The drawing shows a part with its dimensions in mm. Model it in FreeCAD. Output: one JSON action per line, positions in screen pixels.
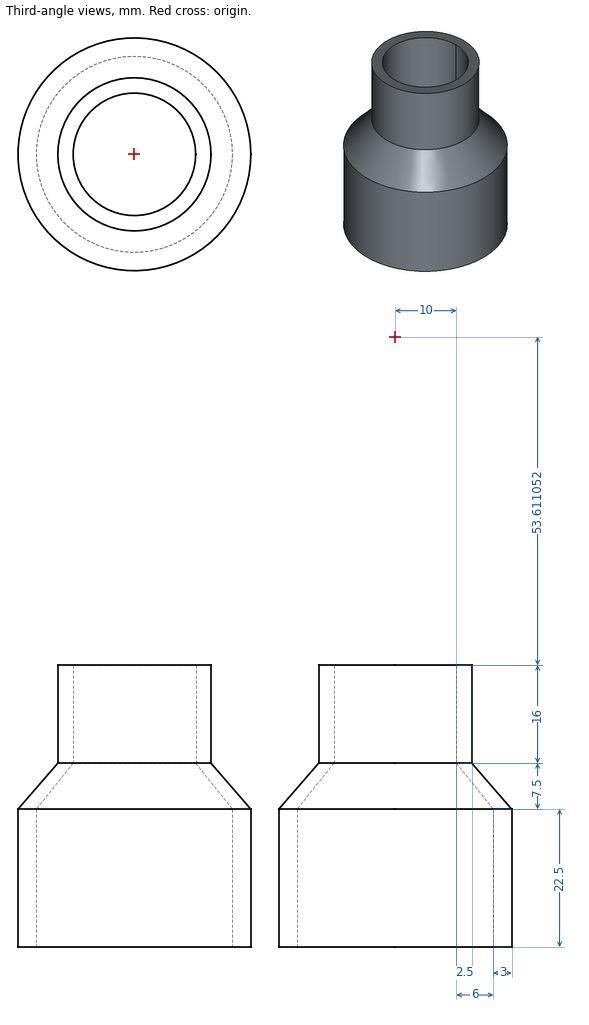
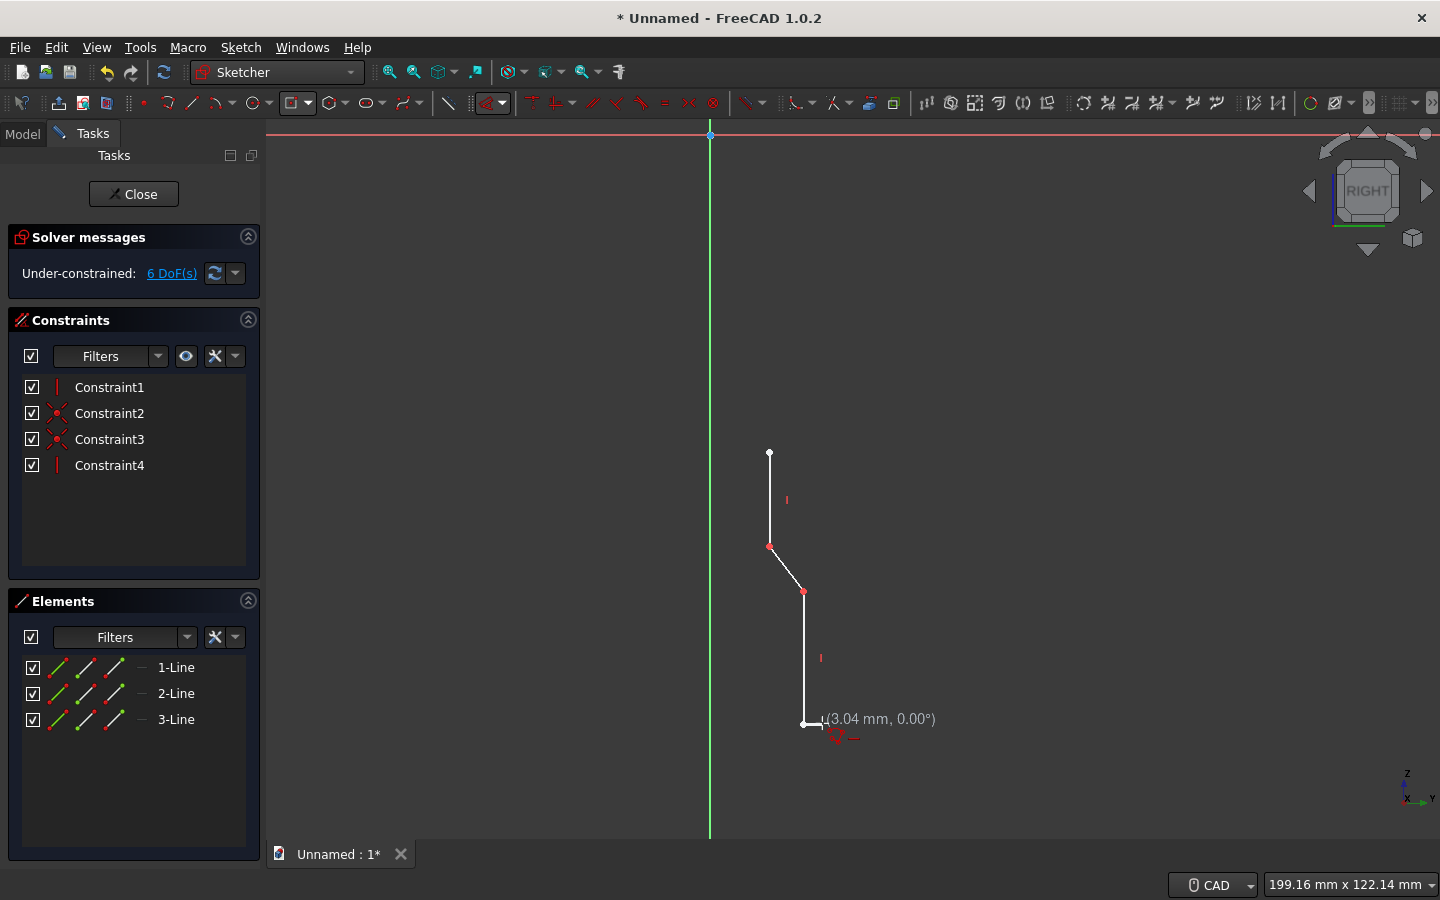
{"action": "left_click", "coordinate": [822, 723]}
{"action": "left_click", "coordinate": [822, 590]}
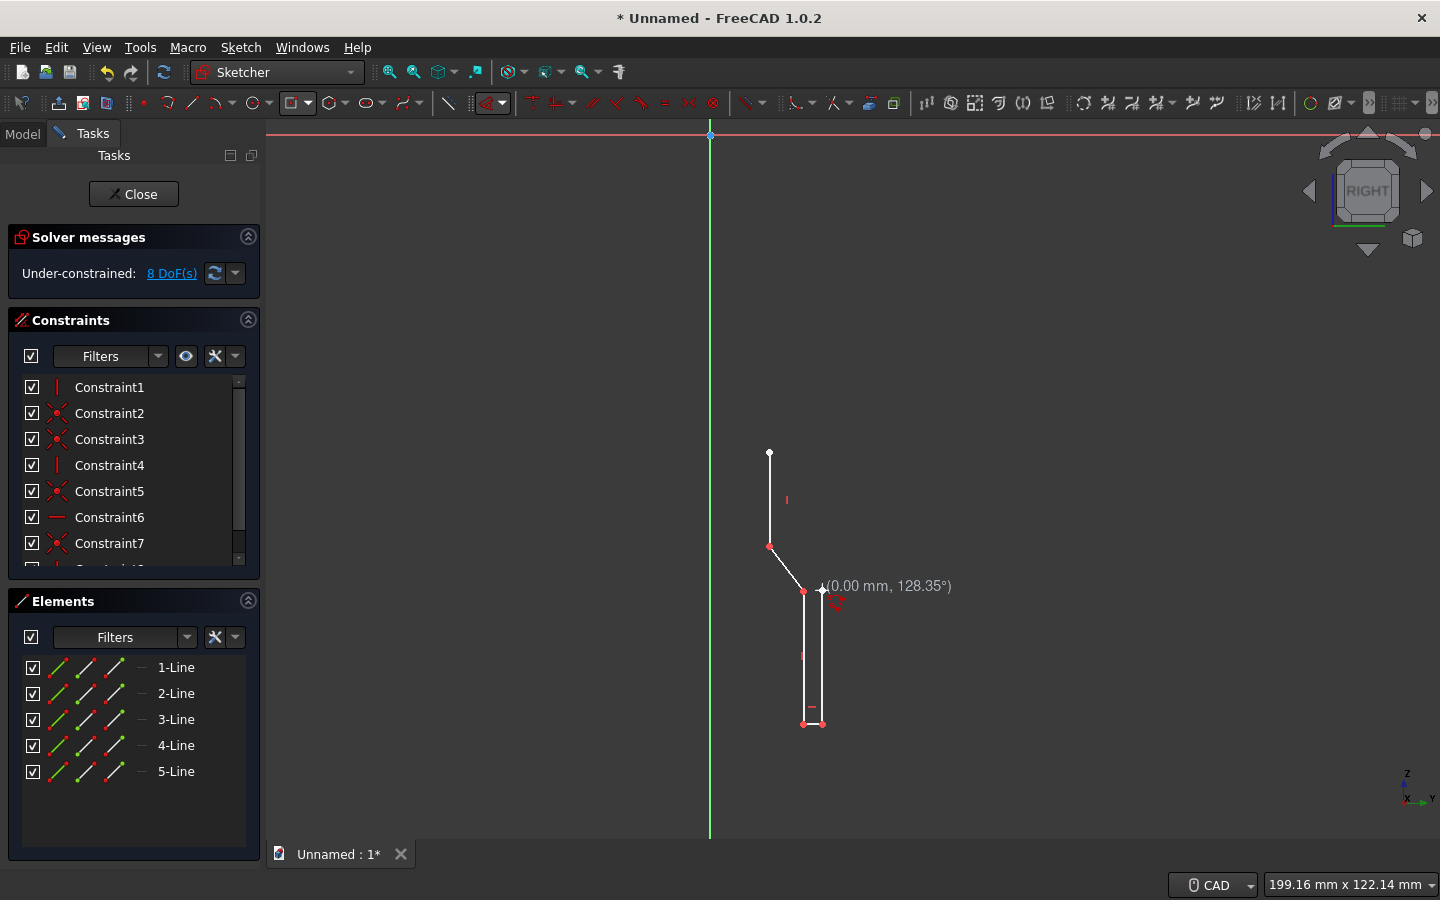
{"action": "scroll", "coordinate": [784, 545], "scroll_direction": "up", "scroll_amount": 2}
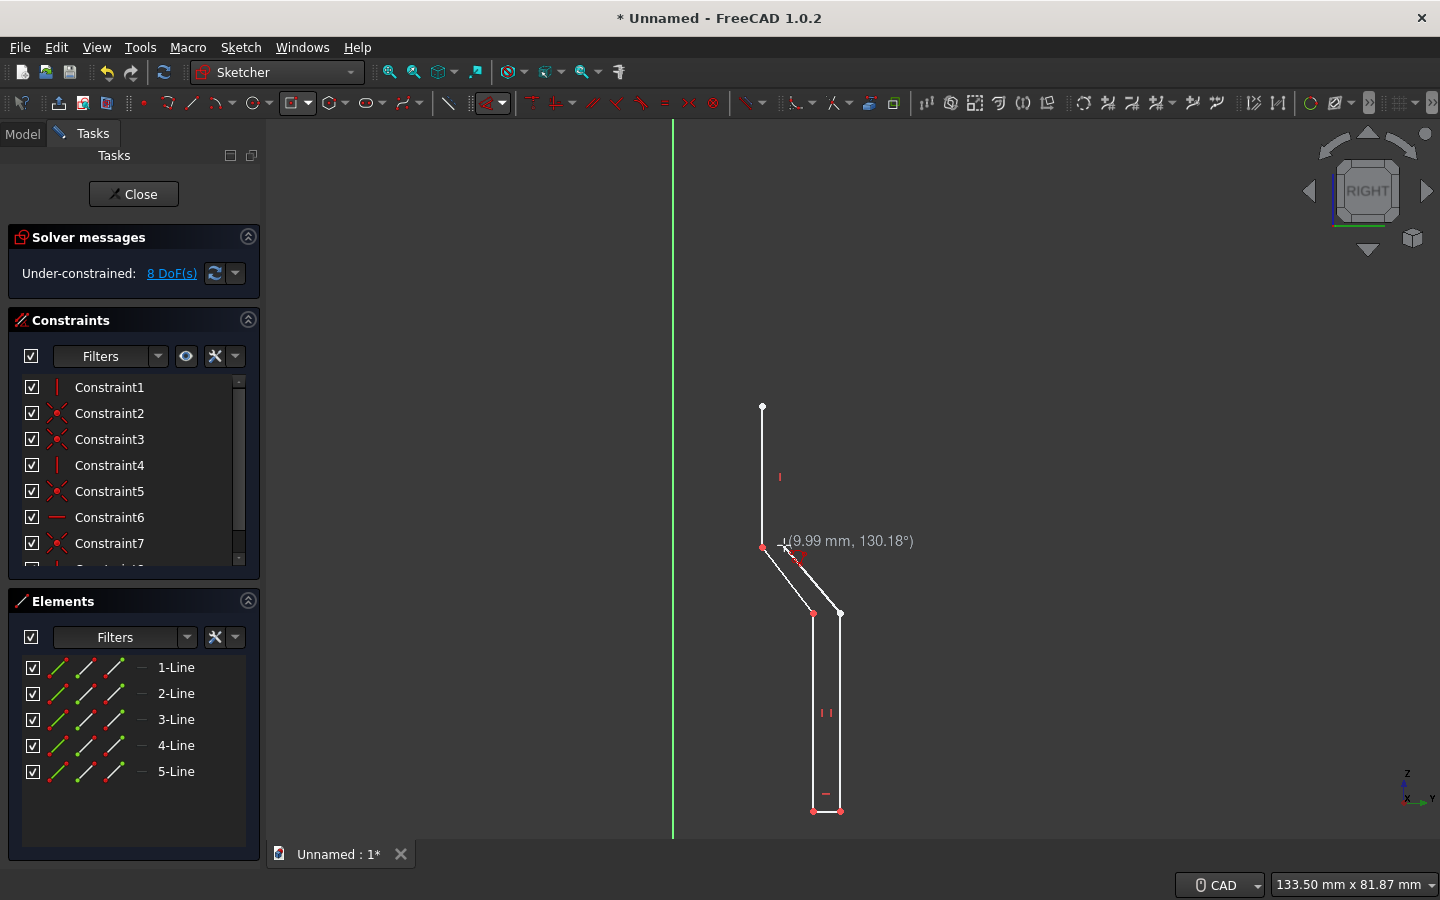
{"action": "left_click", "coordinate": [783, 545]}
{"action": "left_click", "coordinate": [783, 405]}
{"action": "left_click", "coordinate": [762, 407]}
{"action": "key", "text": "Escape"}
{"action": "key", "text": "Escape"}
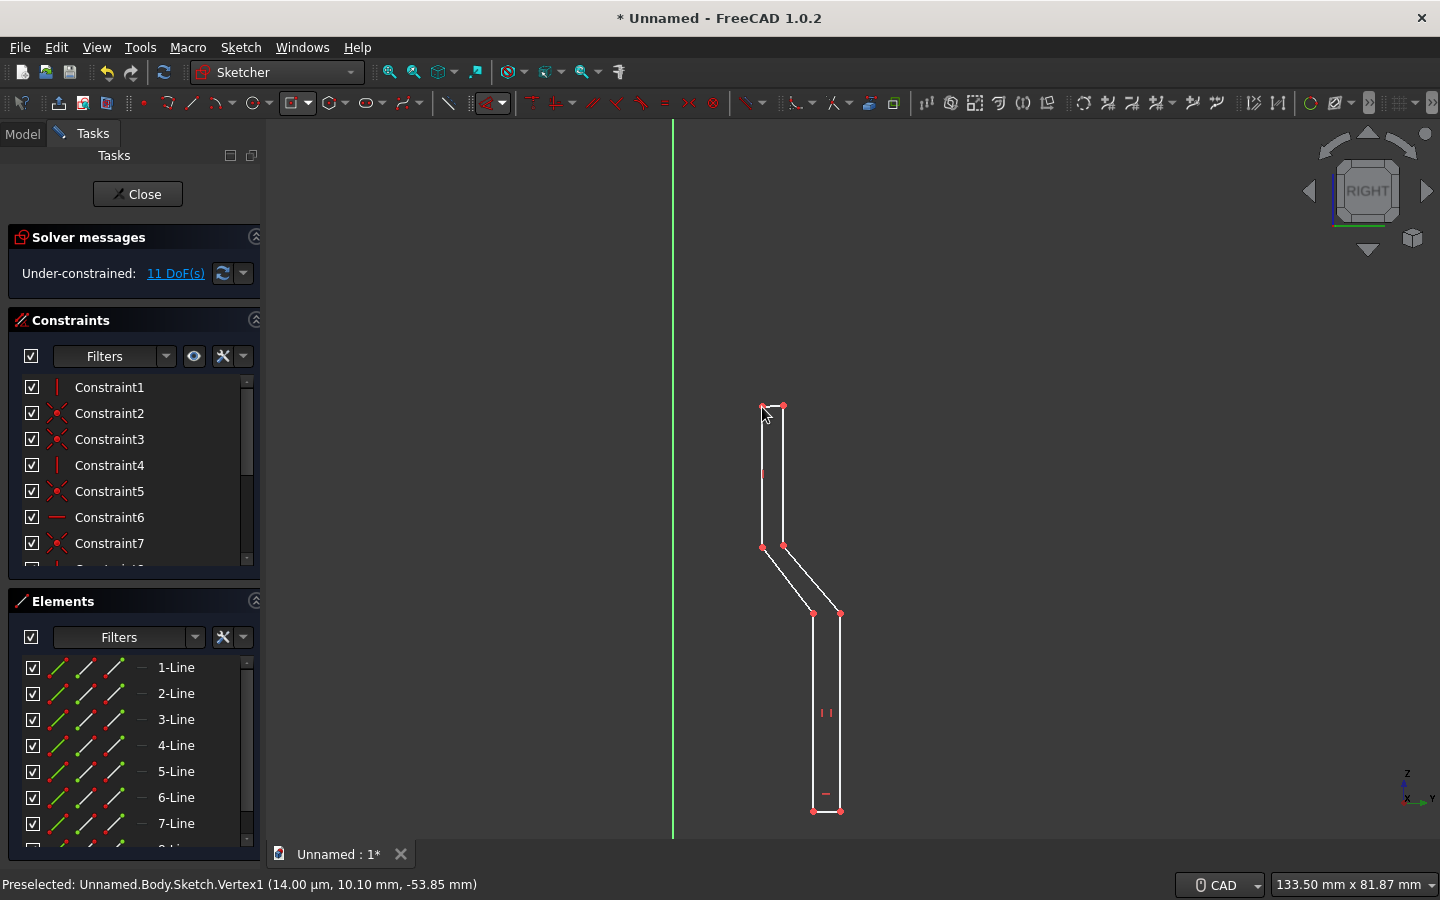
{"action": "scroll", "coordinate": [773, 406], "scroll_direction": "up", "scroll_amount": 2}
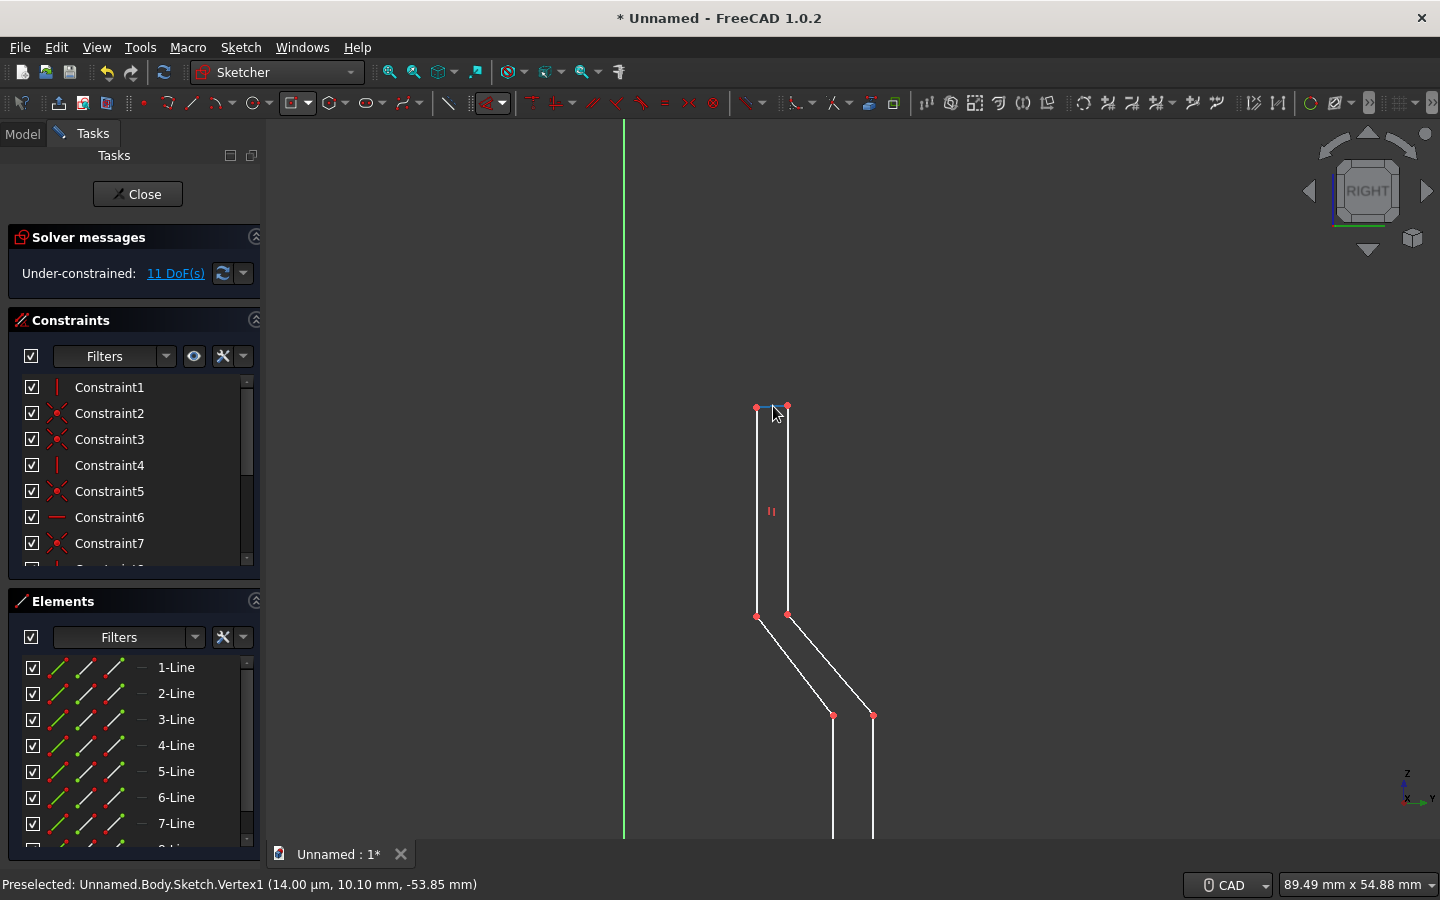
{"action": "left_click", "coordinate": [772, 406]}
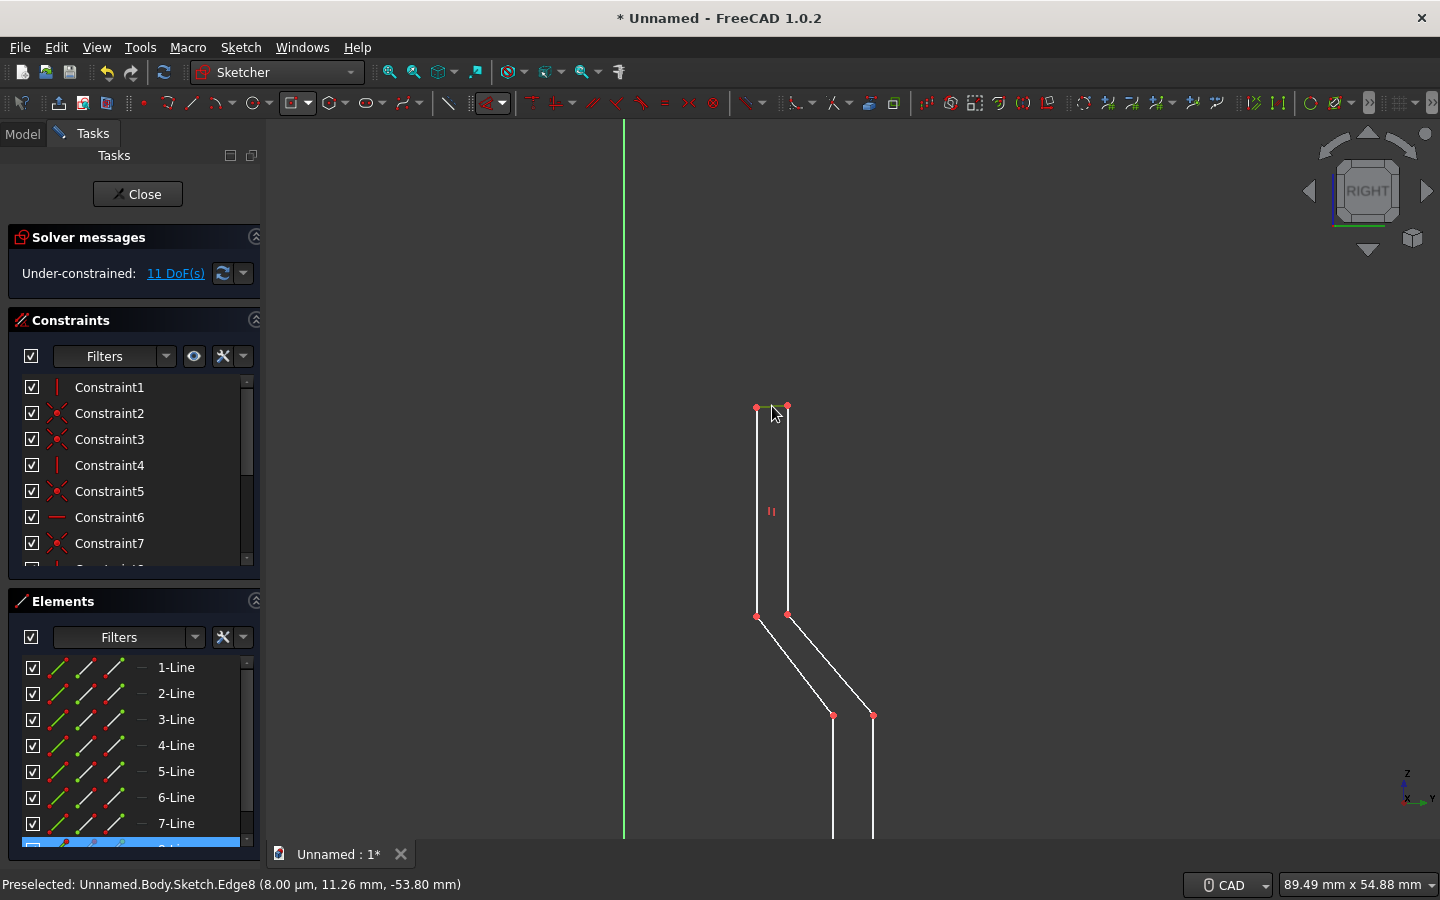
{"action": "left_click", "coordinate": [574, 104]}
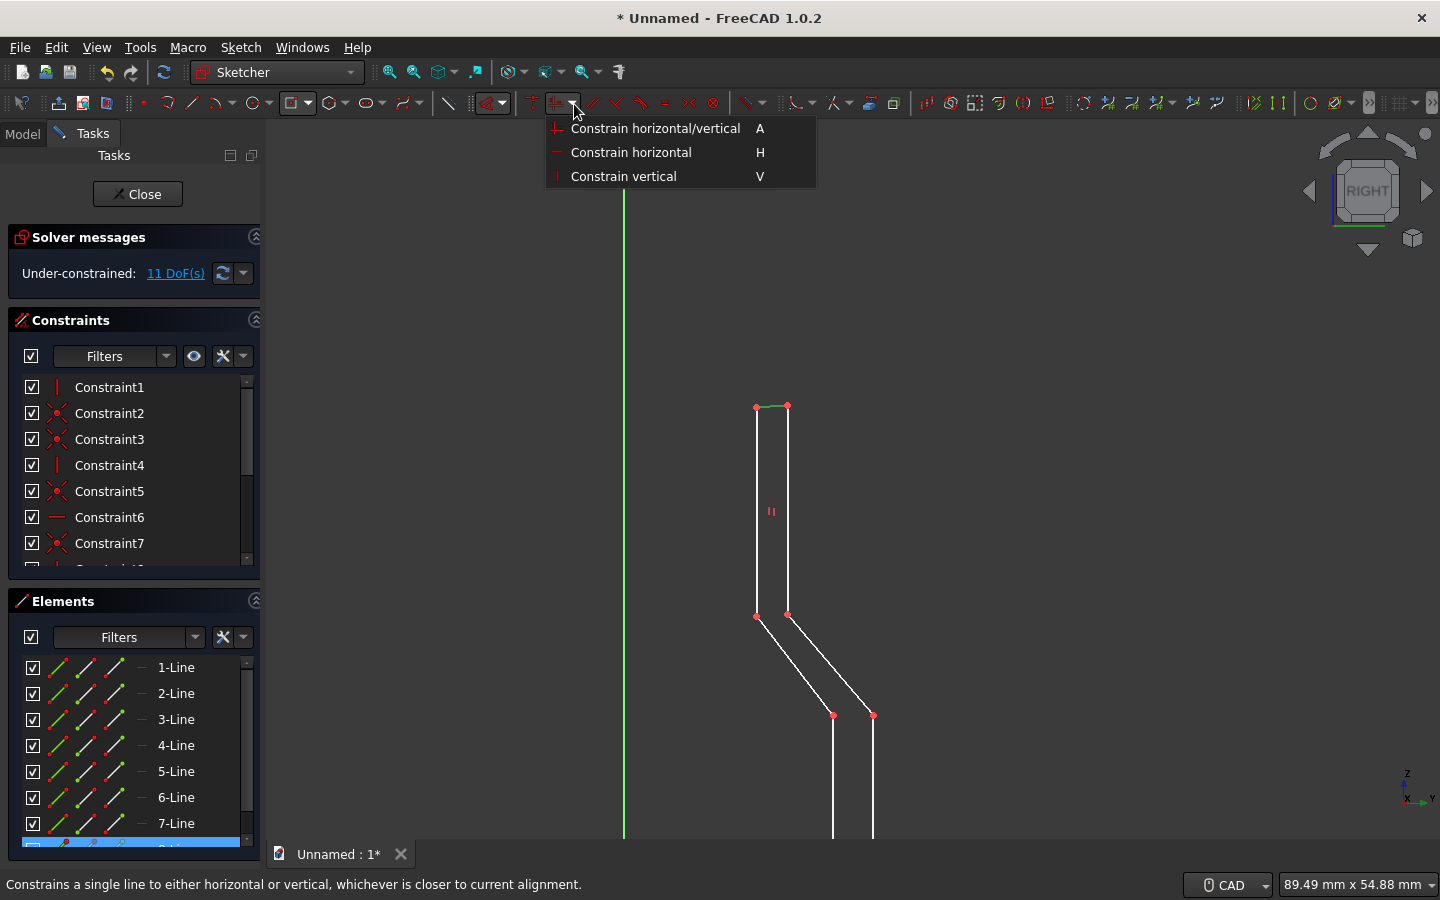
{"action": "left_click", "coordinate": [681, 152]}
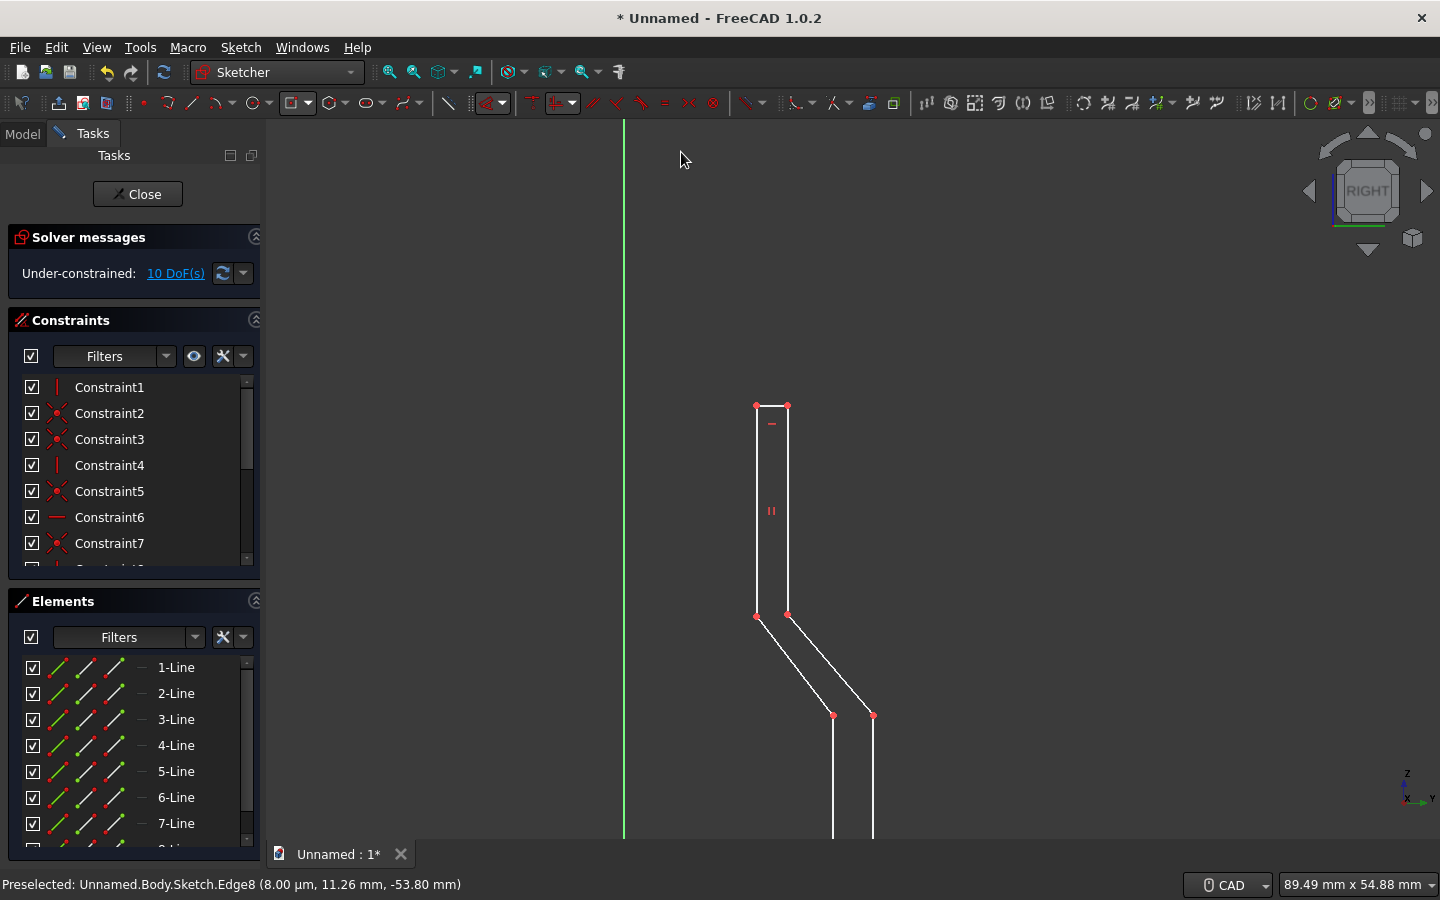
{"action": "left_click", "coordinate": [486, 104]}